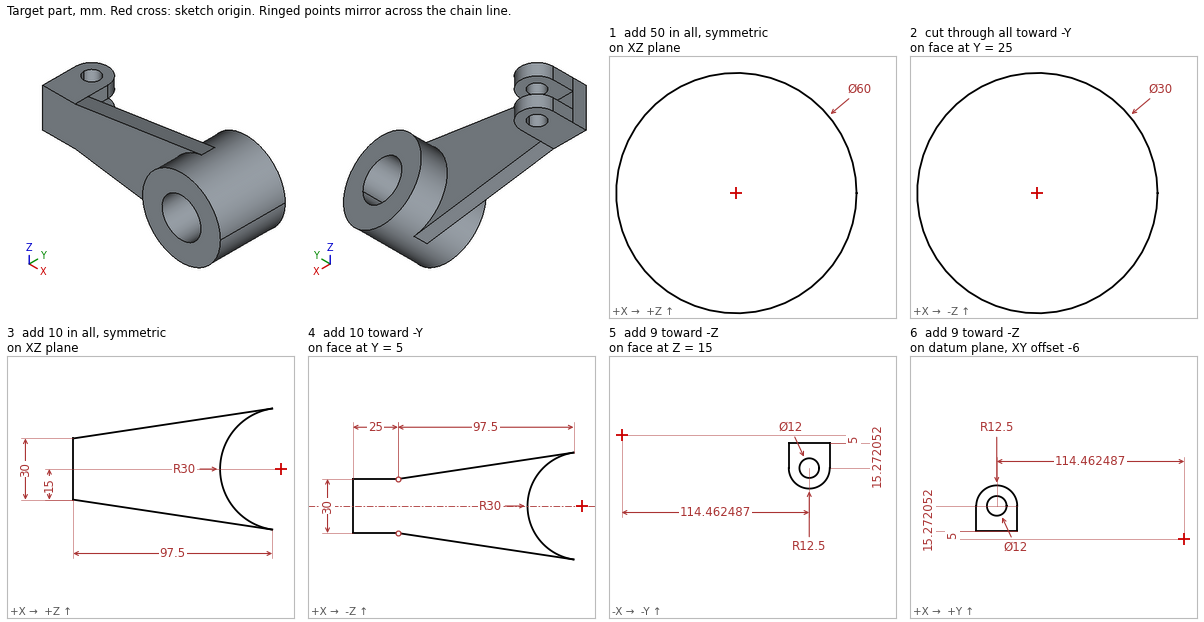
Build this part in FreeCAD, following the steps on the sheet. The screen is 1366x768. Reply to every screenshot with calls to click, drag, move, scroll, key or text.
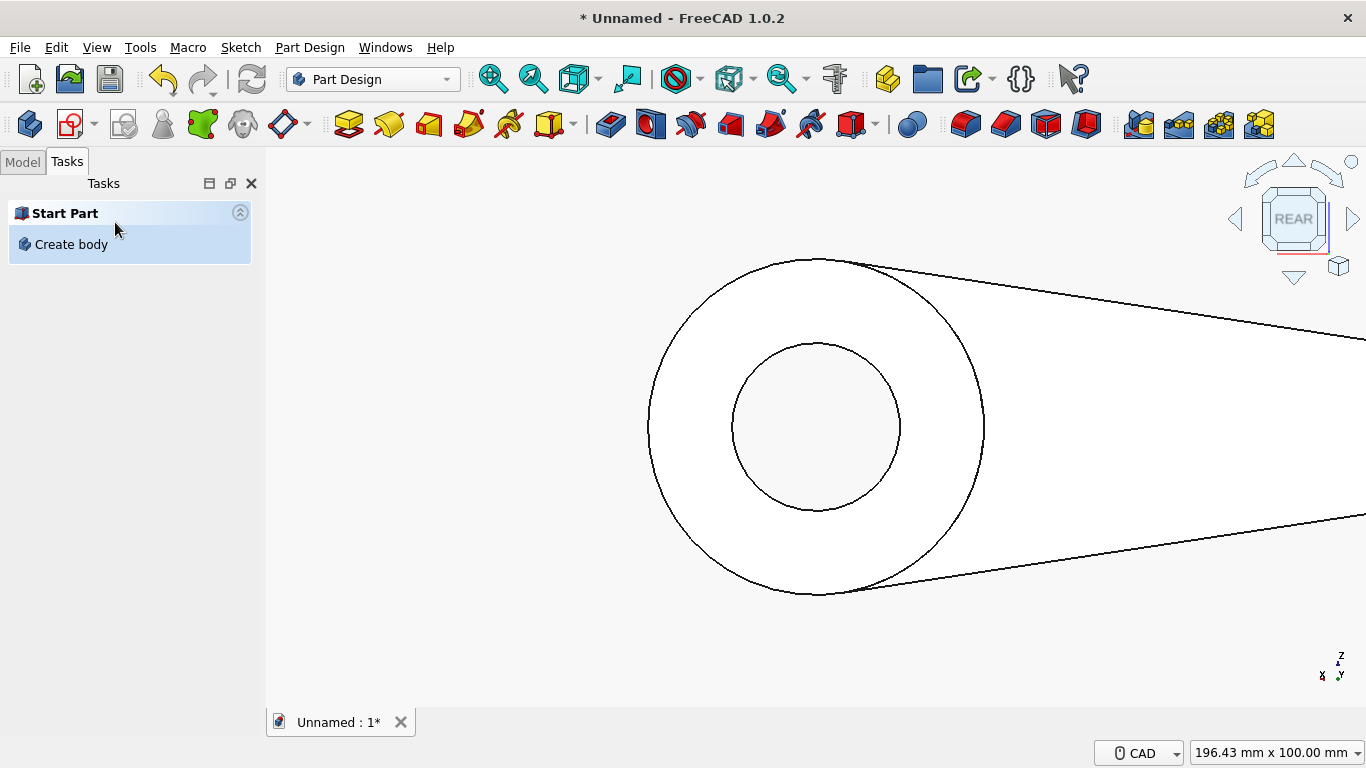
click(494, 80)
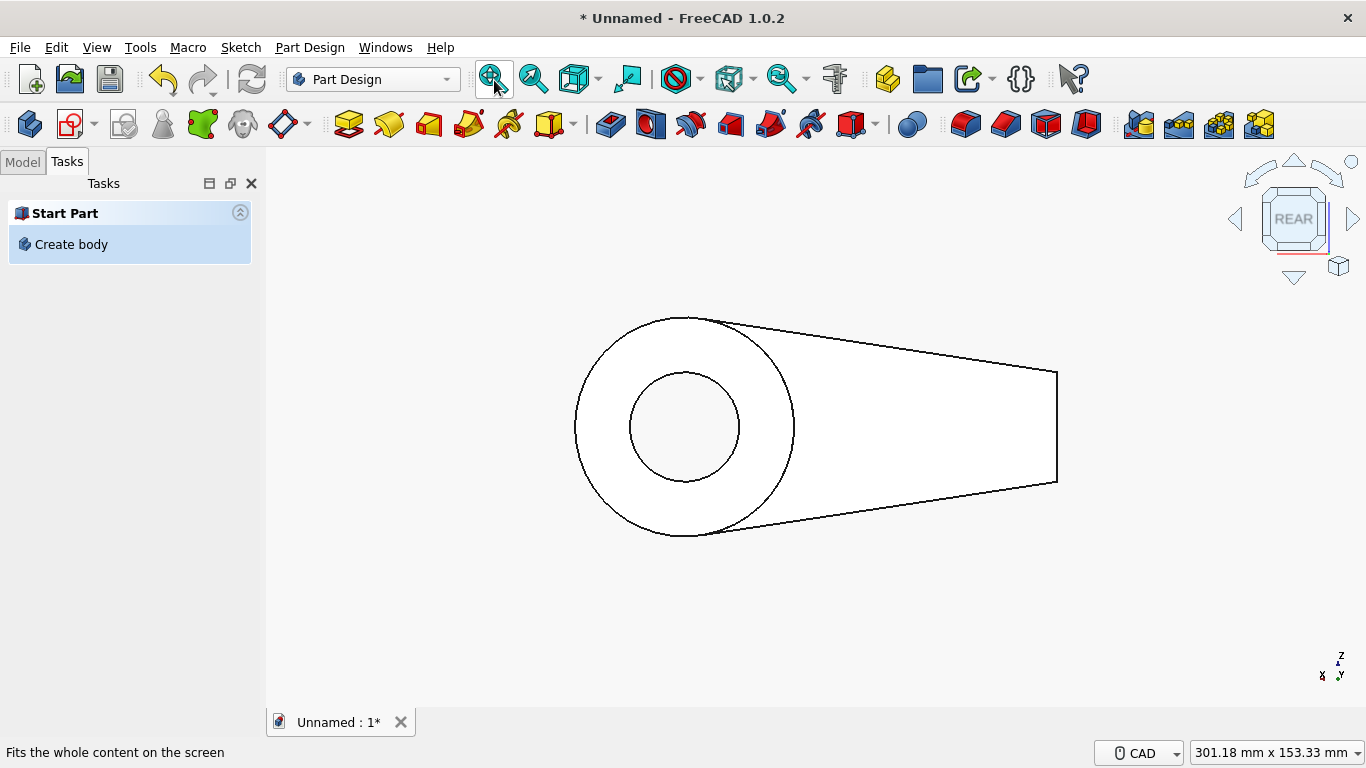
click(879, 426)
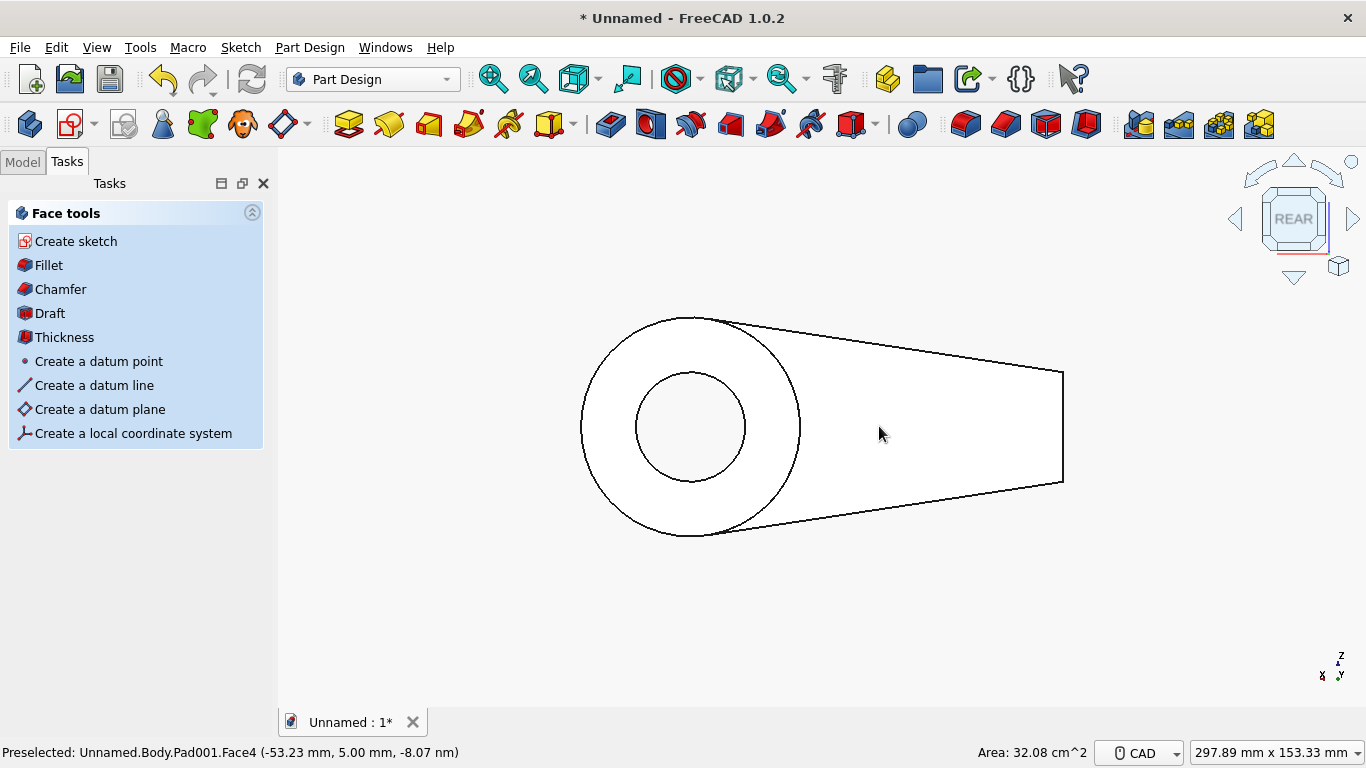
click(70, 124)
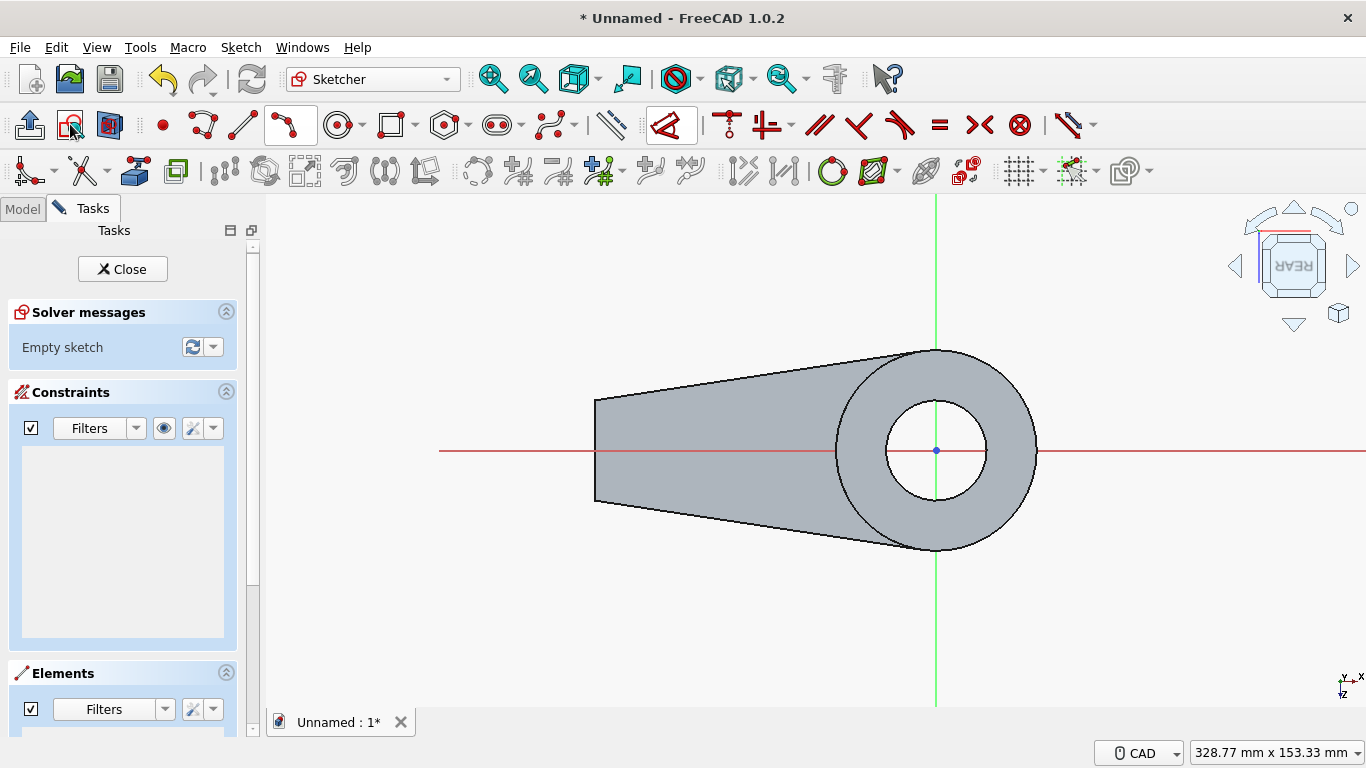
click(110, 126)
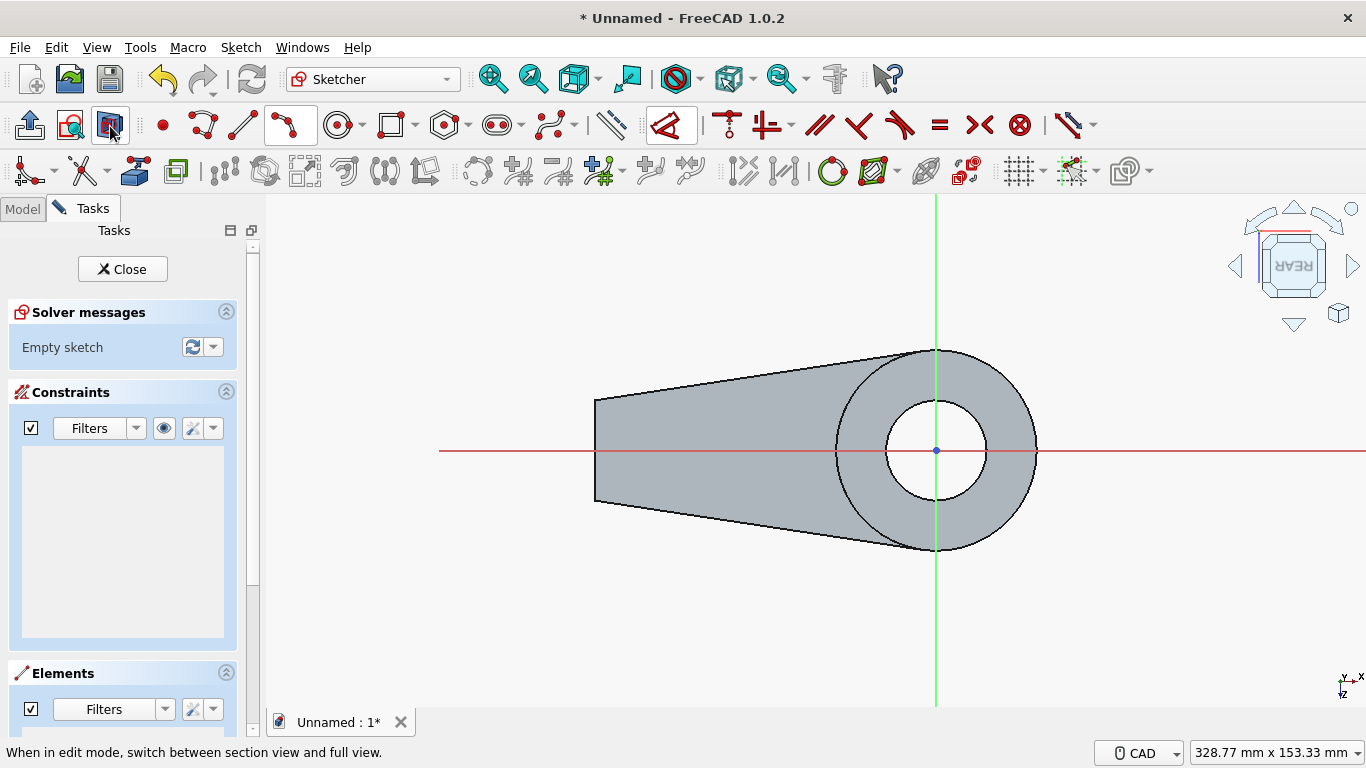
scroll(676, 451, up, 2)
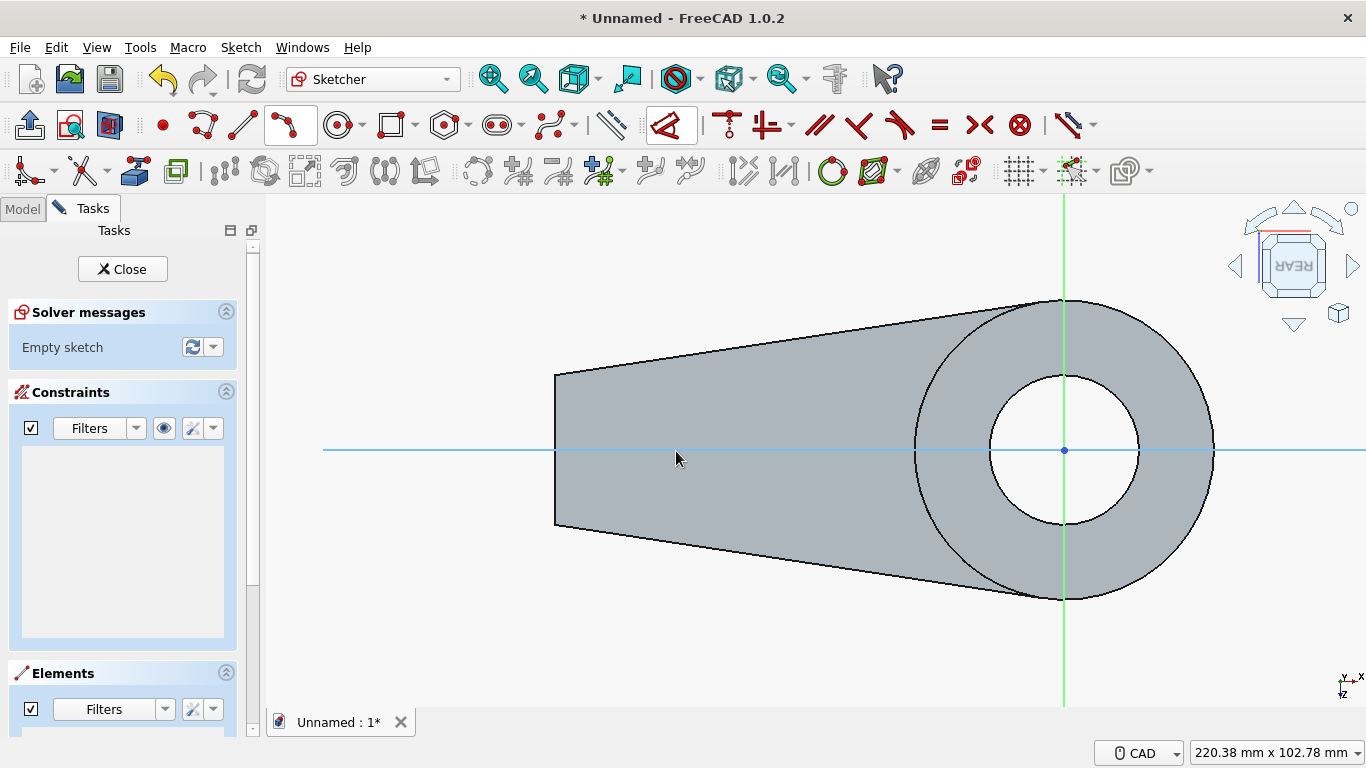
click(204, 126)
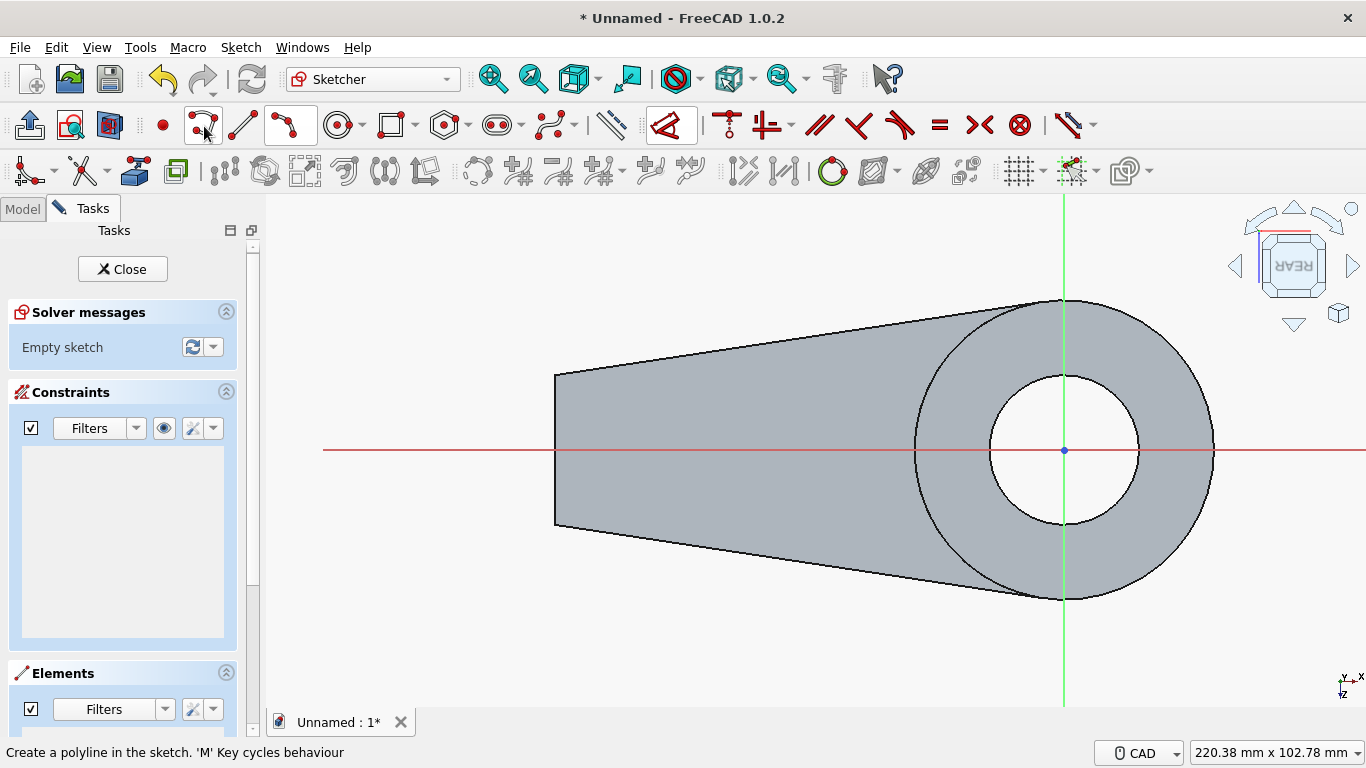
click(1042, 302)
click(555, 375)
click(431, 375)
click(431, 525)
click(555, 525)
click(1042, 598)
right_click(1042, 598)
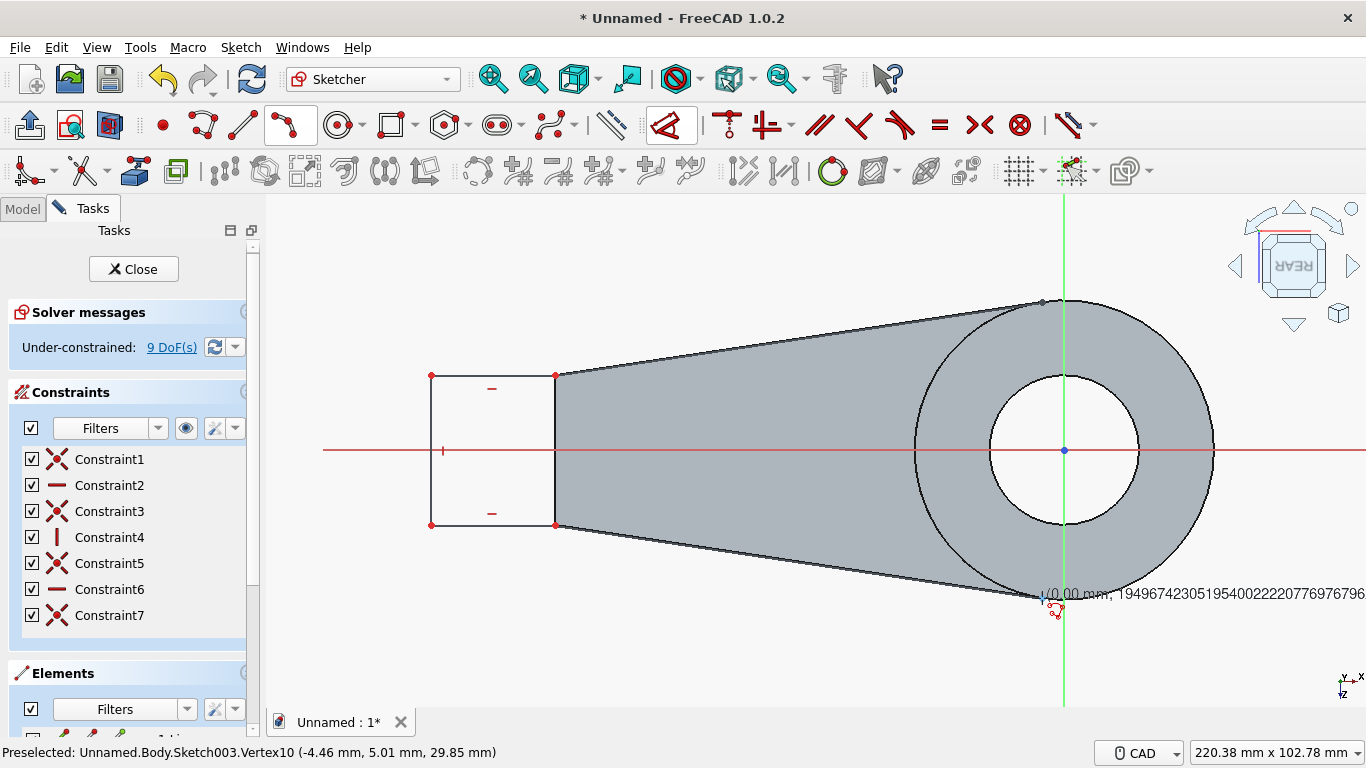
click(284, 126)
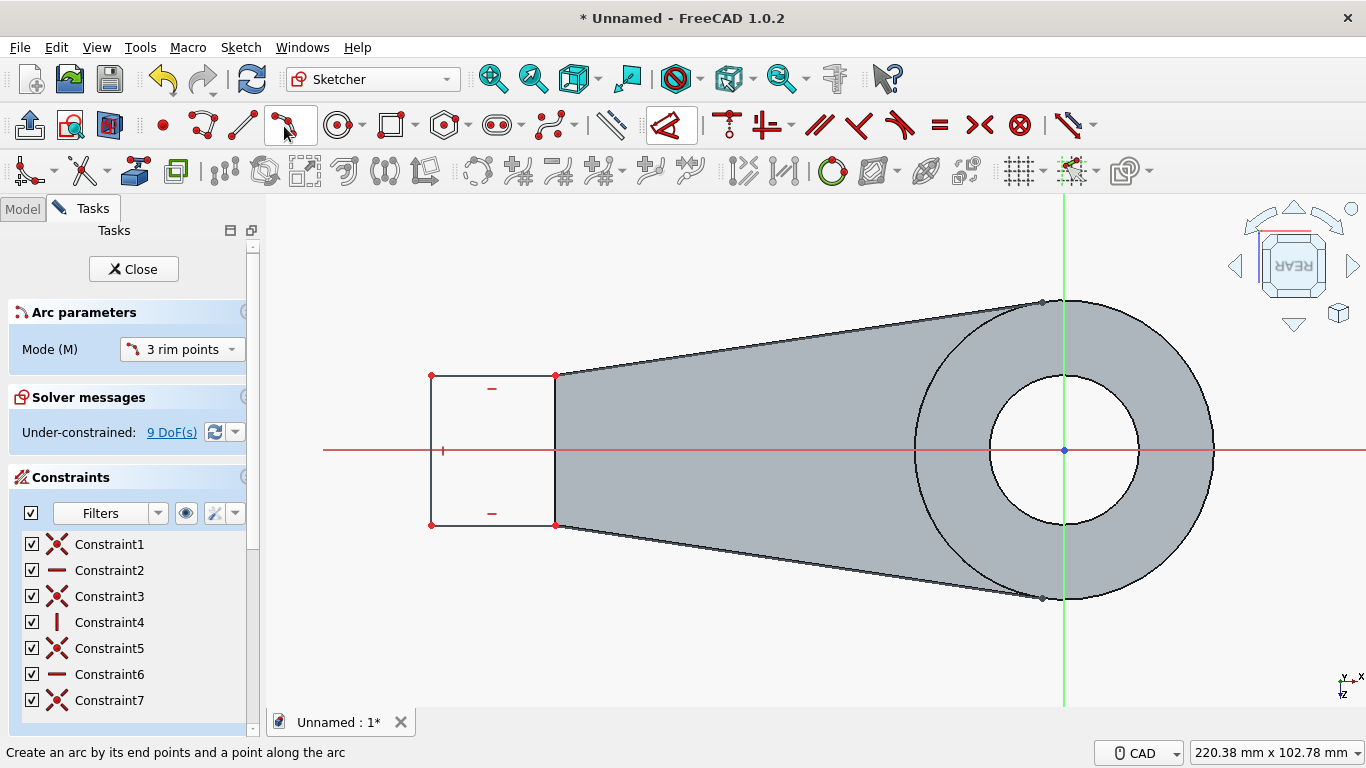
click(1042, 599)
click(1042, 303)
click(921, 408)
key(Escape)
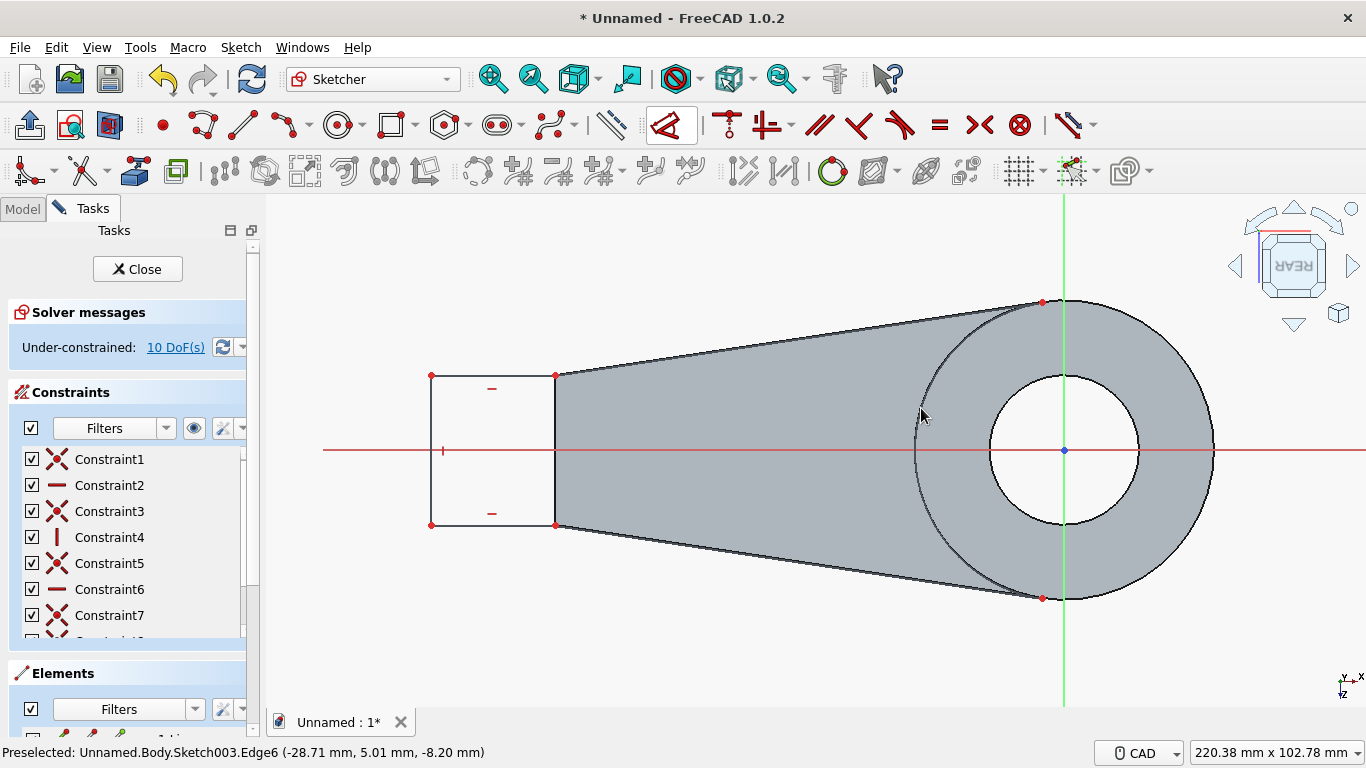
click(896, 325)